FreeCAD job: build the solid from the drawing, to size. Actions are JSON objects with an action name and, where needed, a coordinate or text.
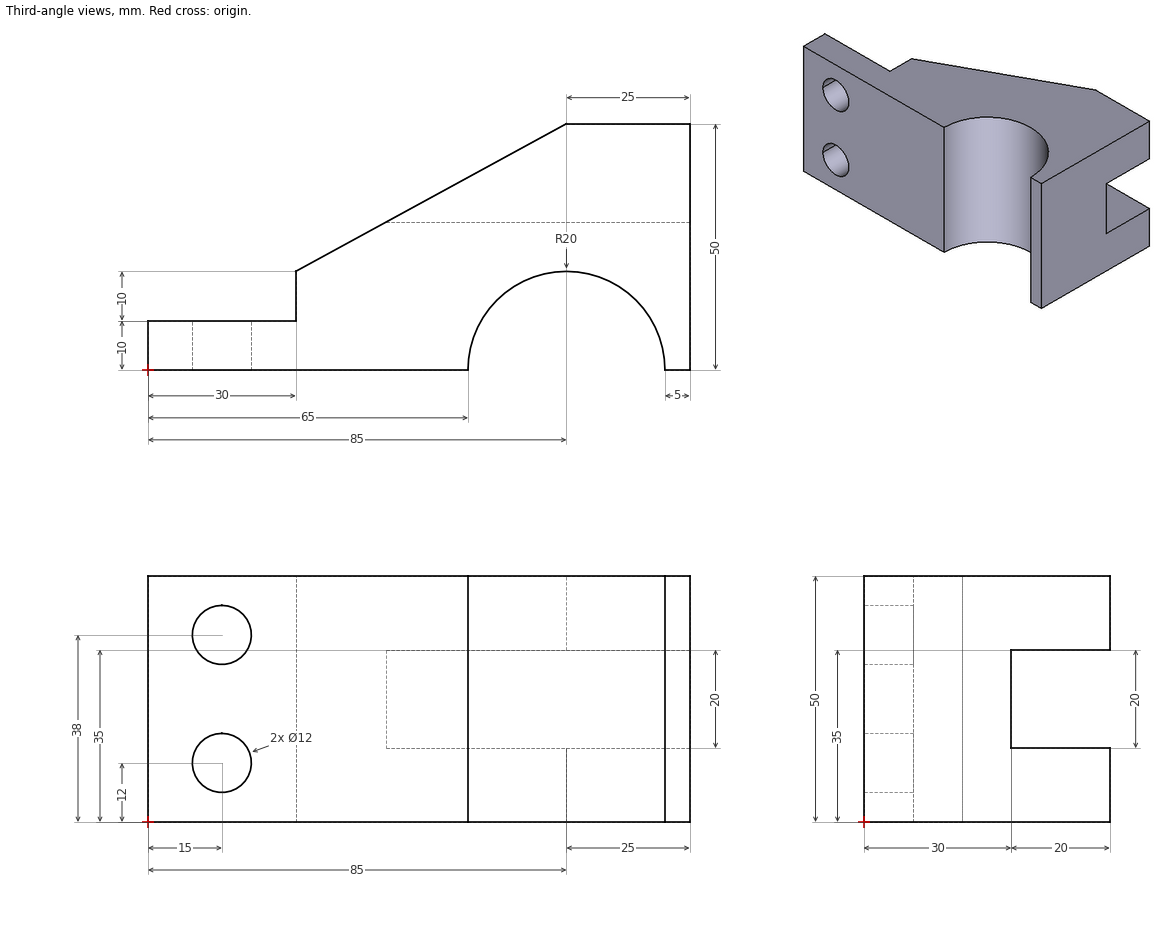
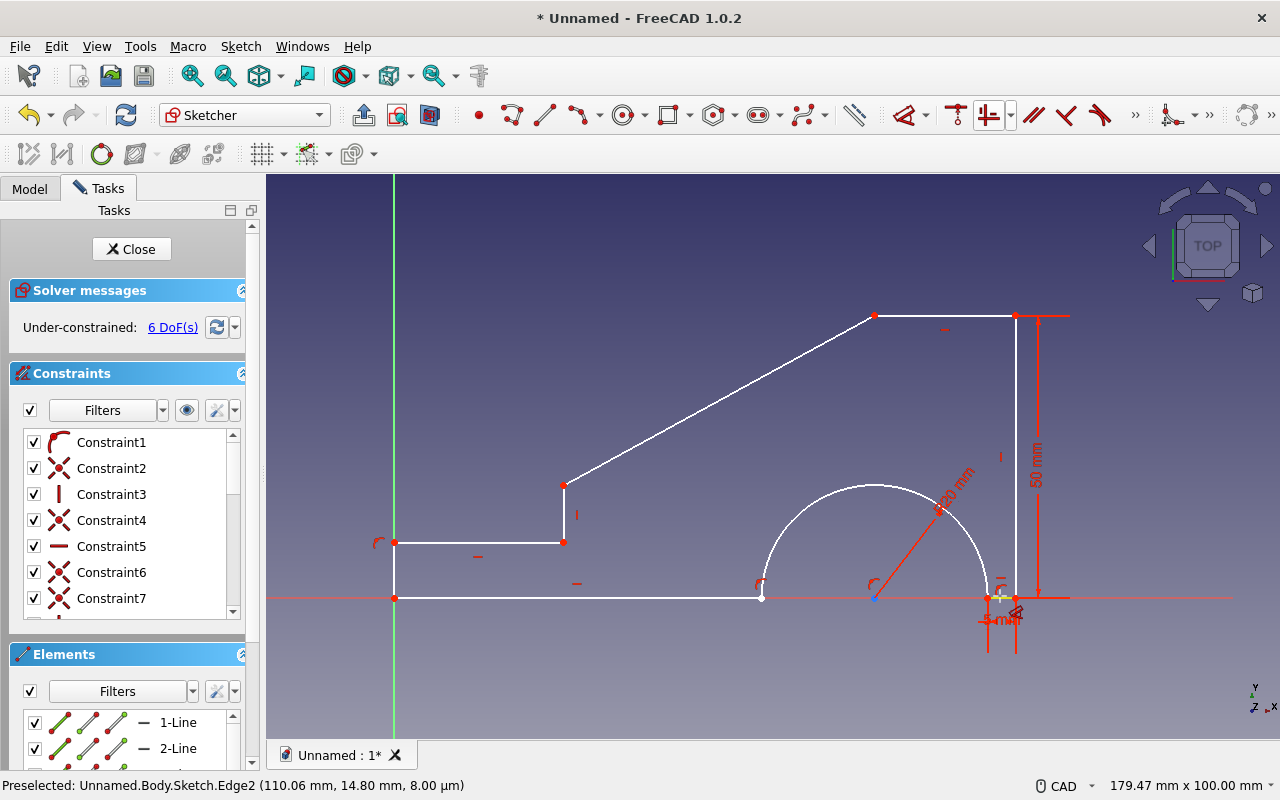
{"action": "left_click", "coordinate": [974, 316]}
{"action": "left_click", "coordinate": [945, 282]}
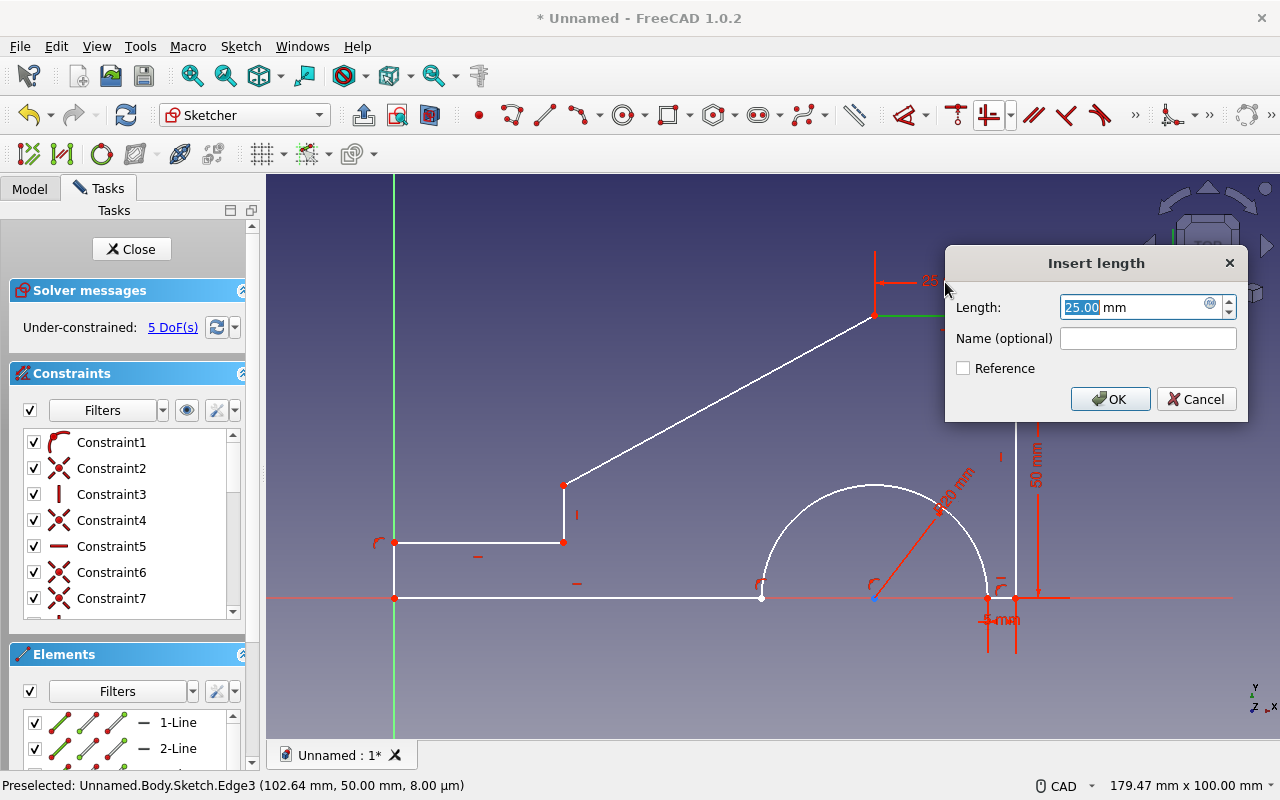
{"action": "type", "text": "25"}
{"action": "key", "text": "Return"}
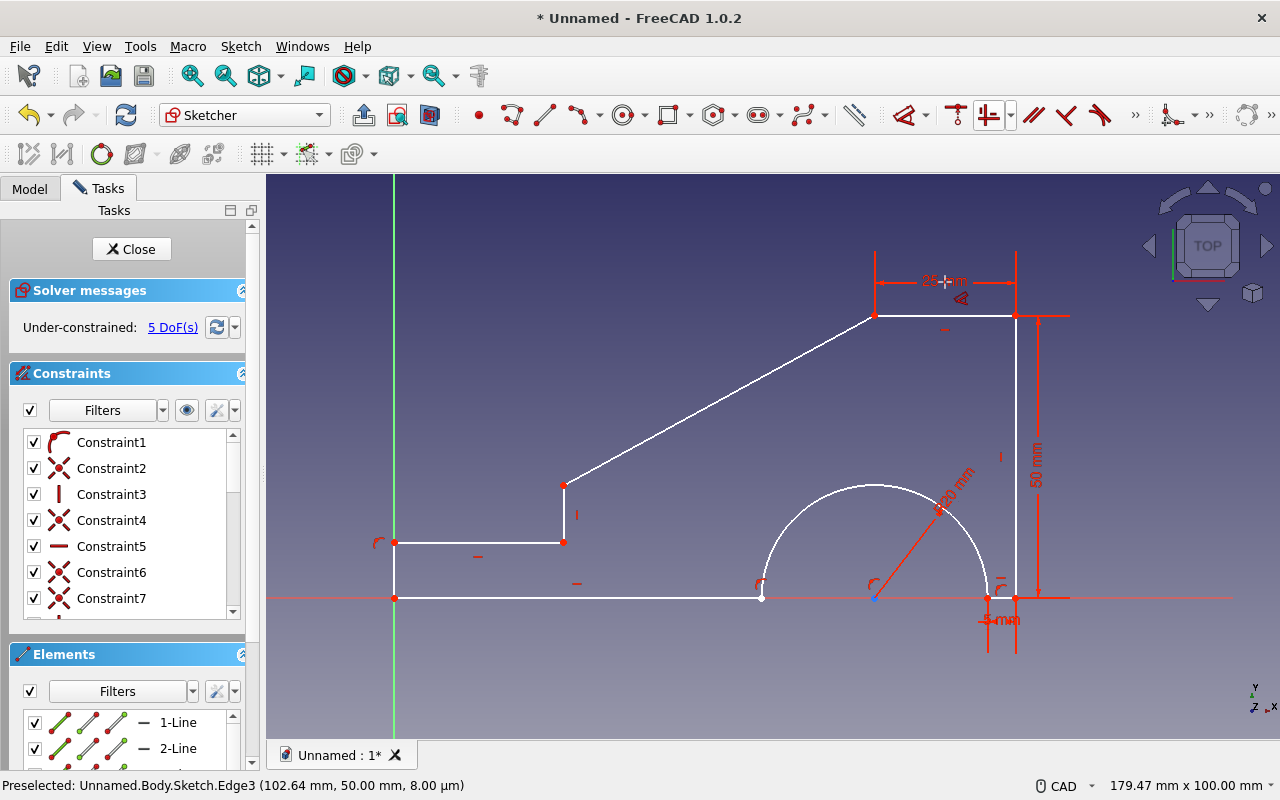
{"action": "left_click", "coordinate": [564, 503]}
{"action": "left_click", "coordinate": [530, 514]}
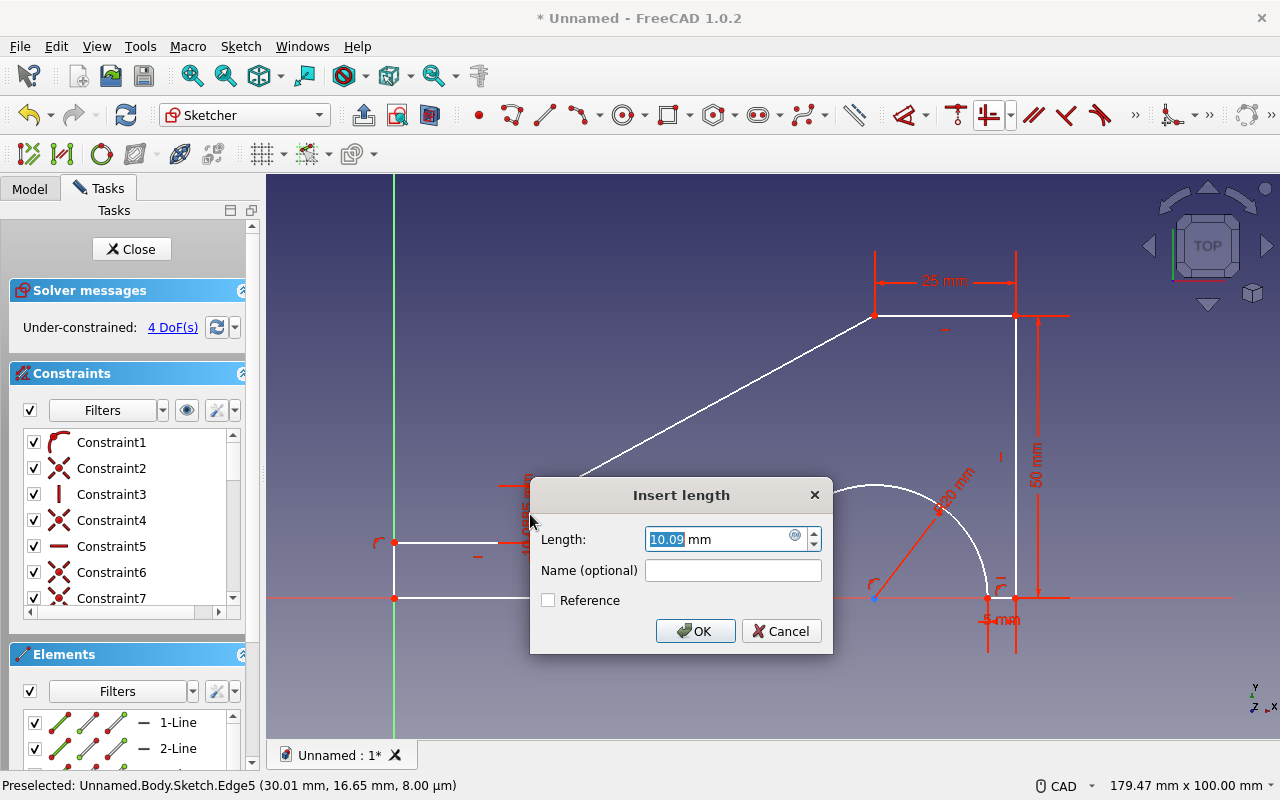
{"action": "type", "text": "10"}
{"action": "key", "text": "Return"}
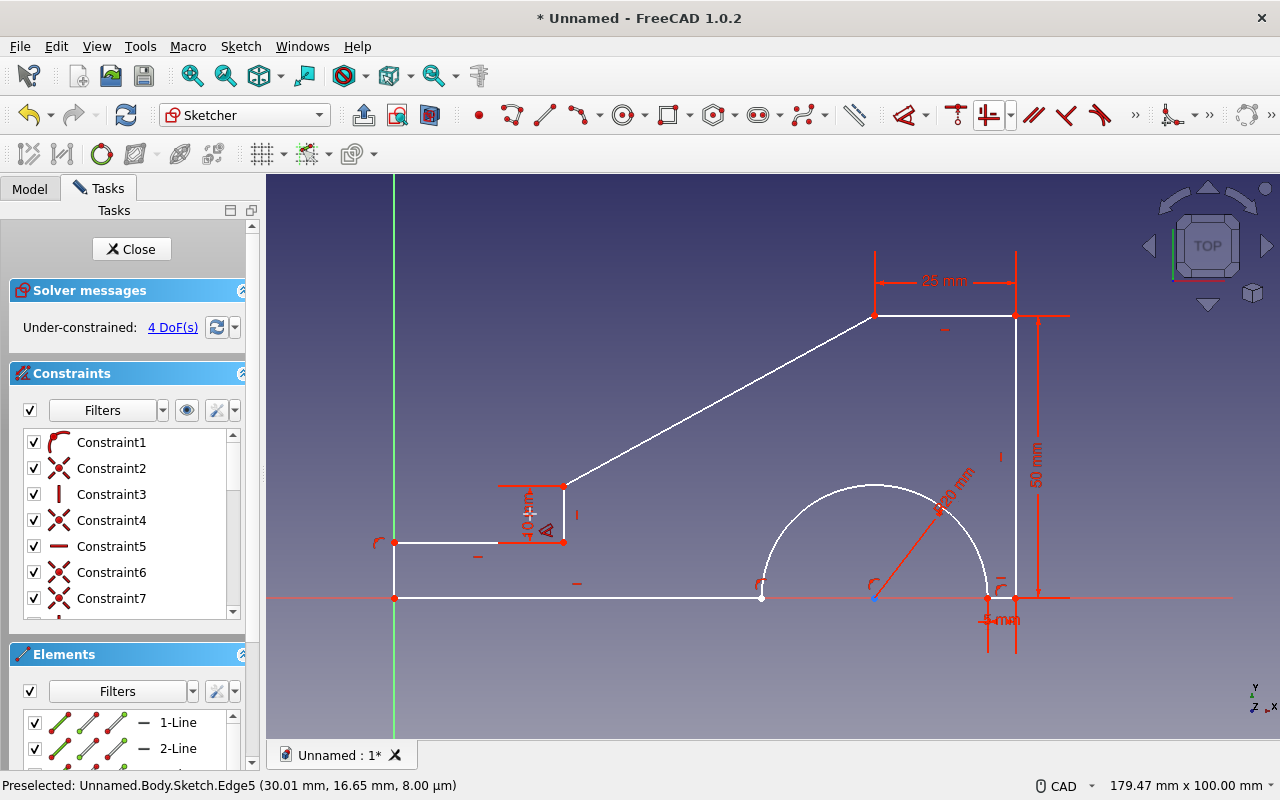
{"action": "left_click", "coordinate": [513, 543]}
{"action": "left_click", "coordinate": [479, 577]}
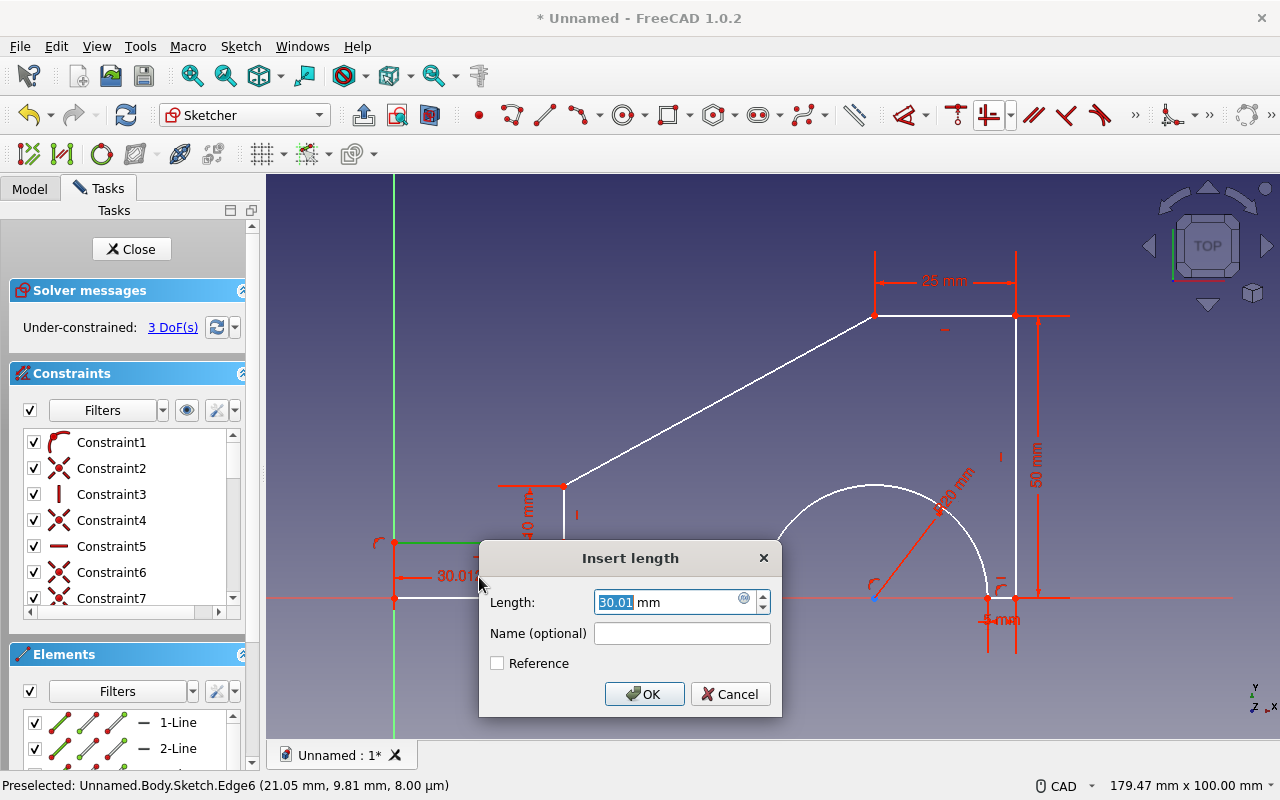
{"action": "type", "text": "30"}
{"action": "key", "text": "Return"}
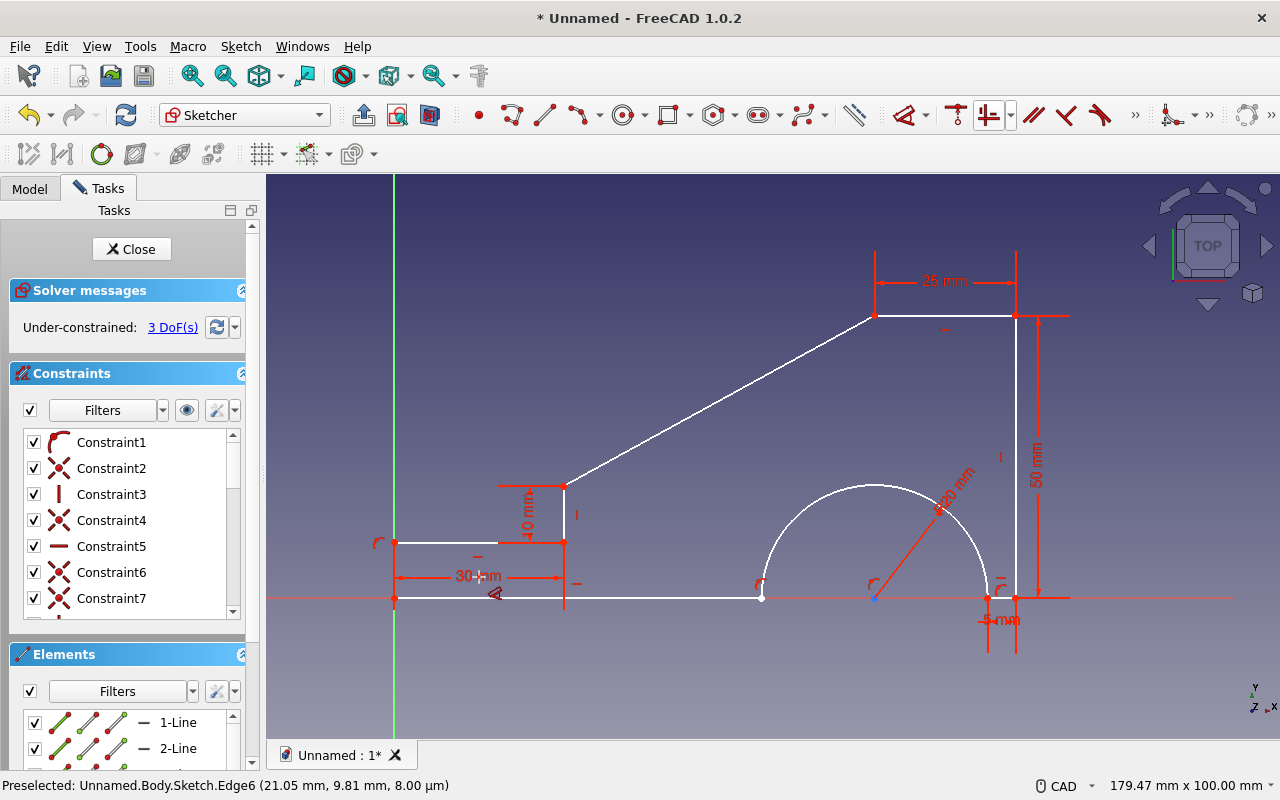
{"action": "left_click", "coordinate": [394, 559]}
{"action": "left_click", "coordinate": [360, 570]}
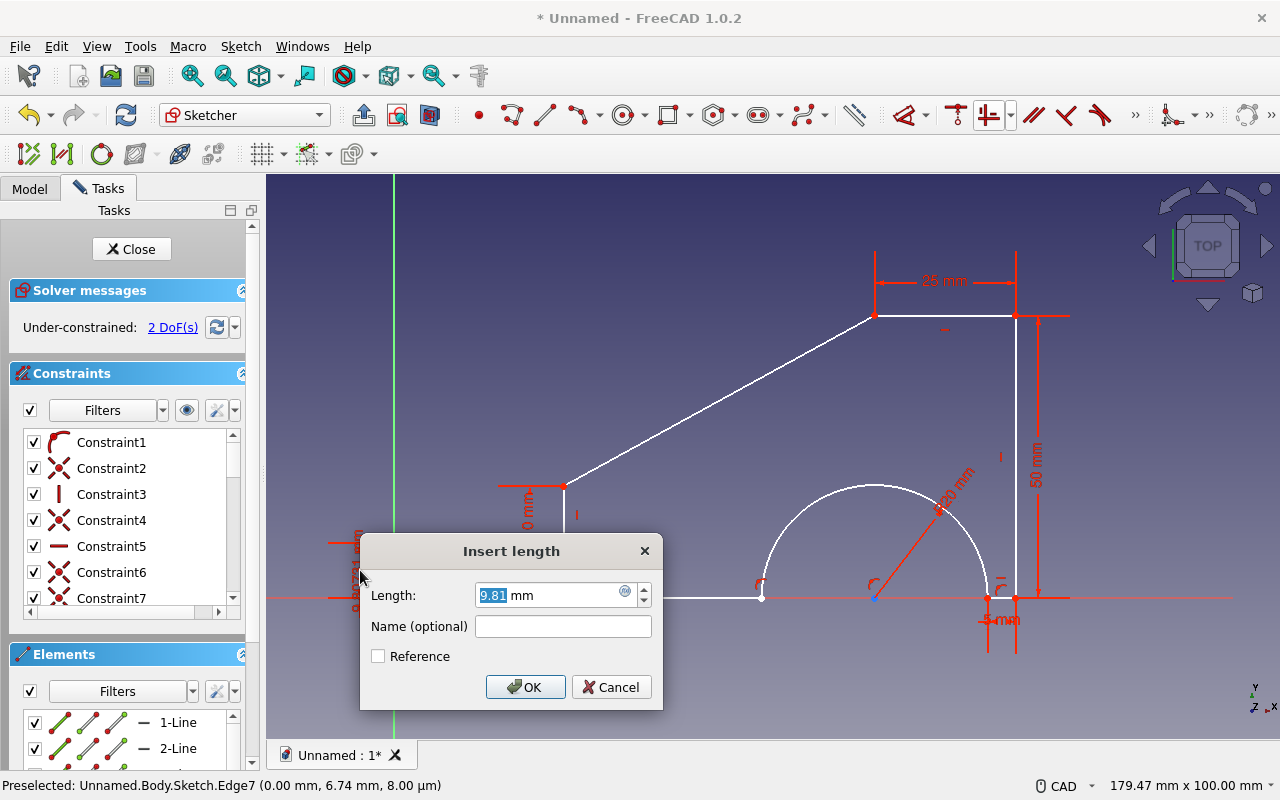
{"action": "type", "text": "10"}
{"action": "key", "text": "Return"}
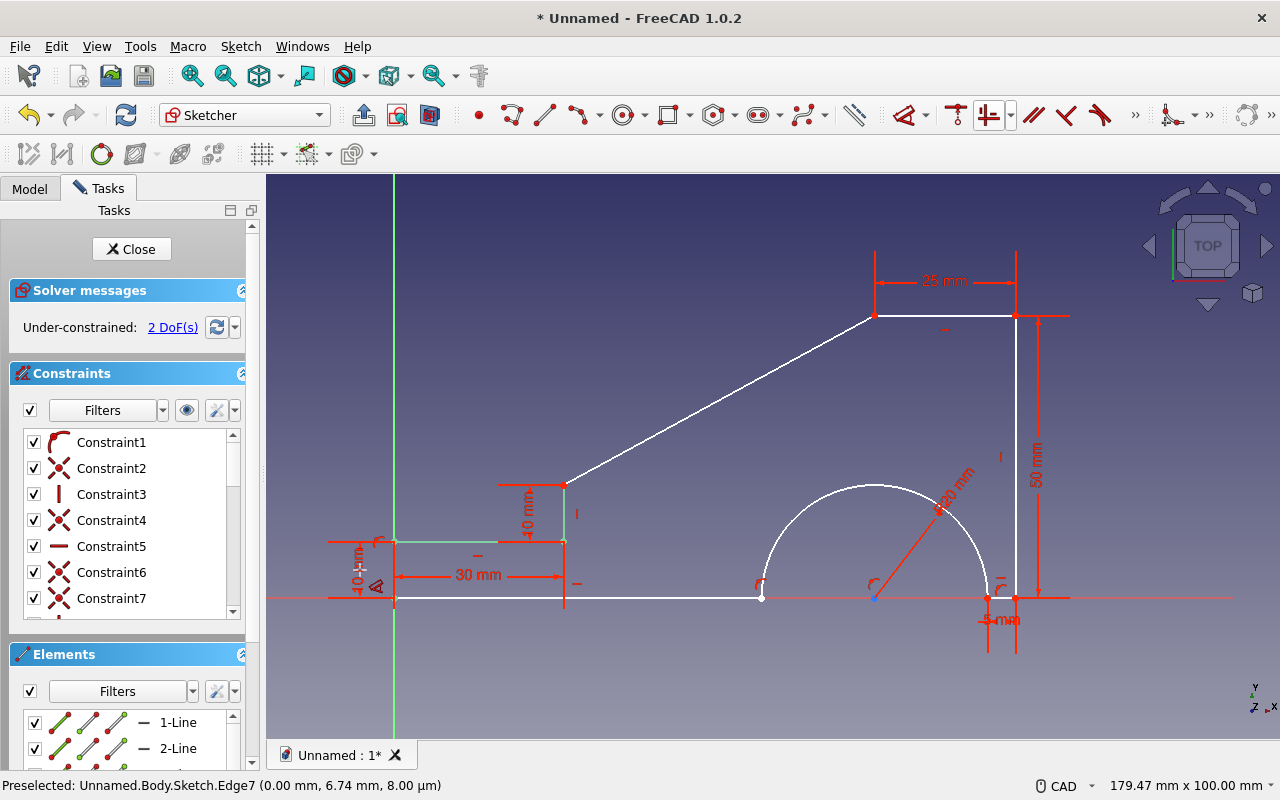
{"action": "left_click", "coordinate": [504, 598]}
{"action": "left_click", "coordinate": [578, 632]}